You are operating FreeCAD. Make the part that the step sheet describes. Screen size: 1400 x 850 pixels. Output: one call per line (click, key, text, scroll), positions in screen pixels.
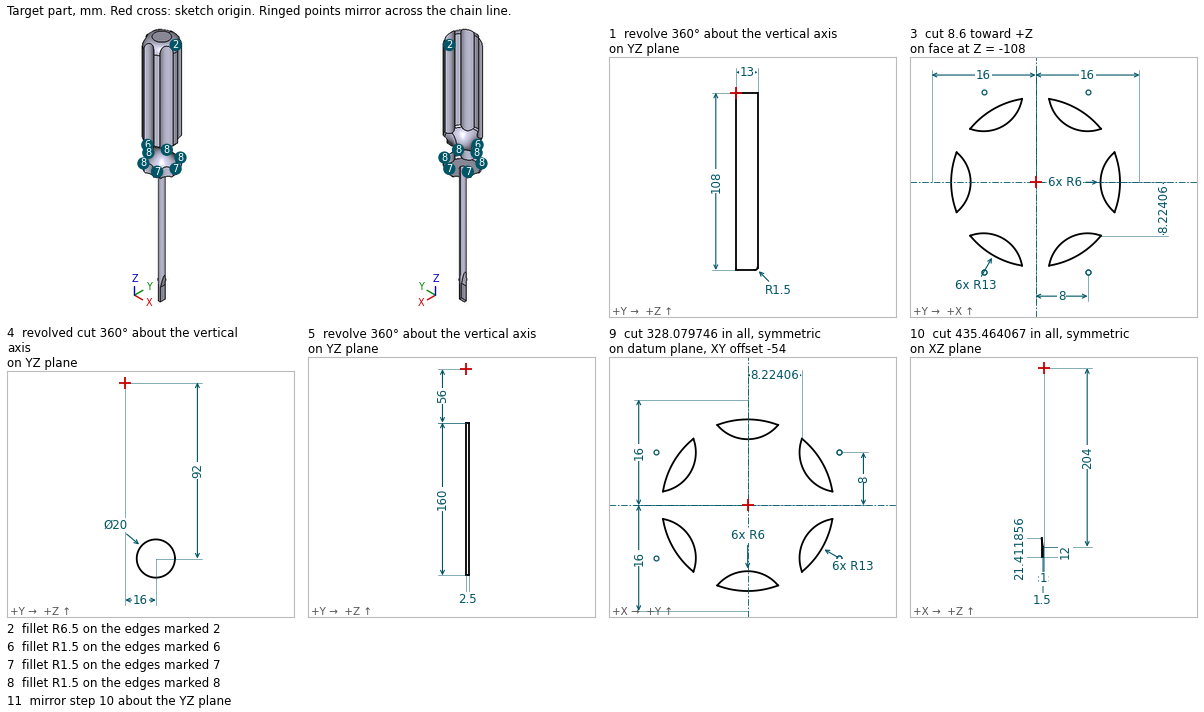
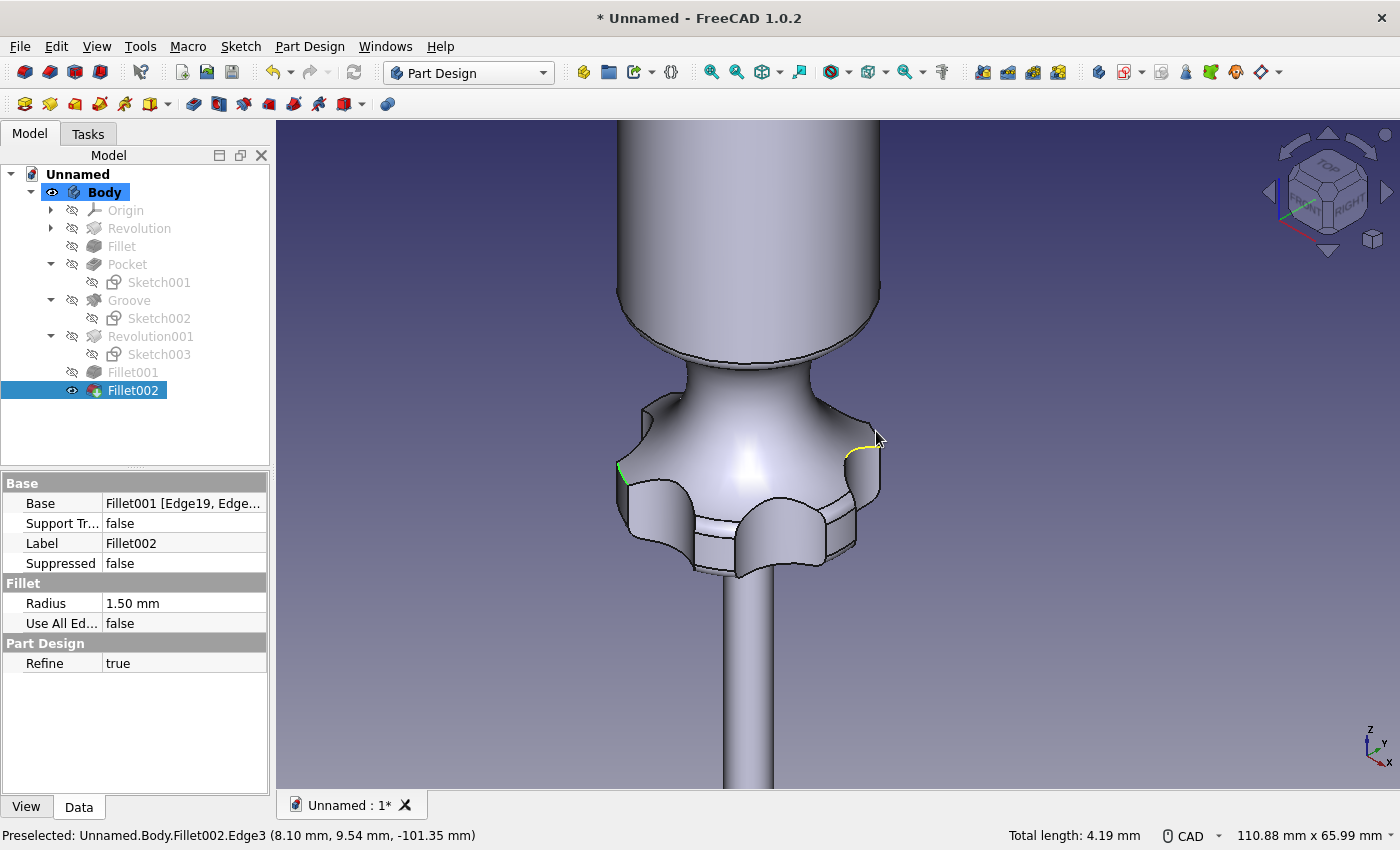
click(712, 72)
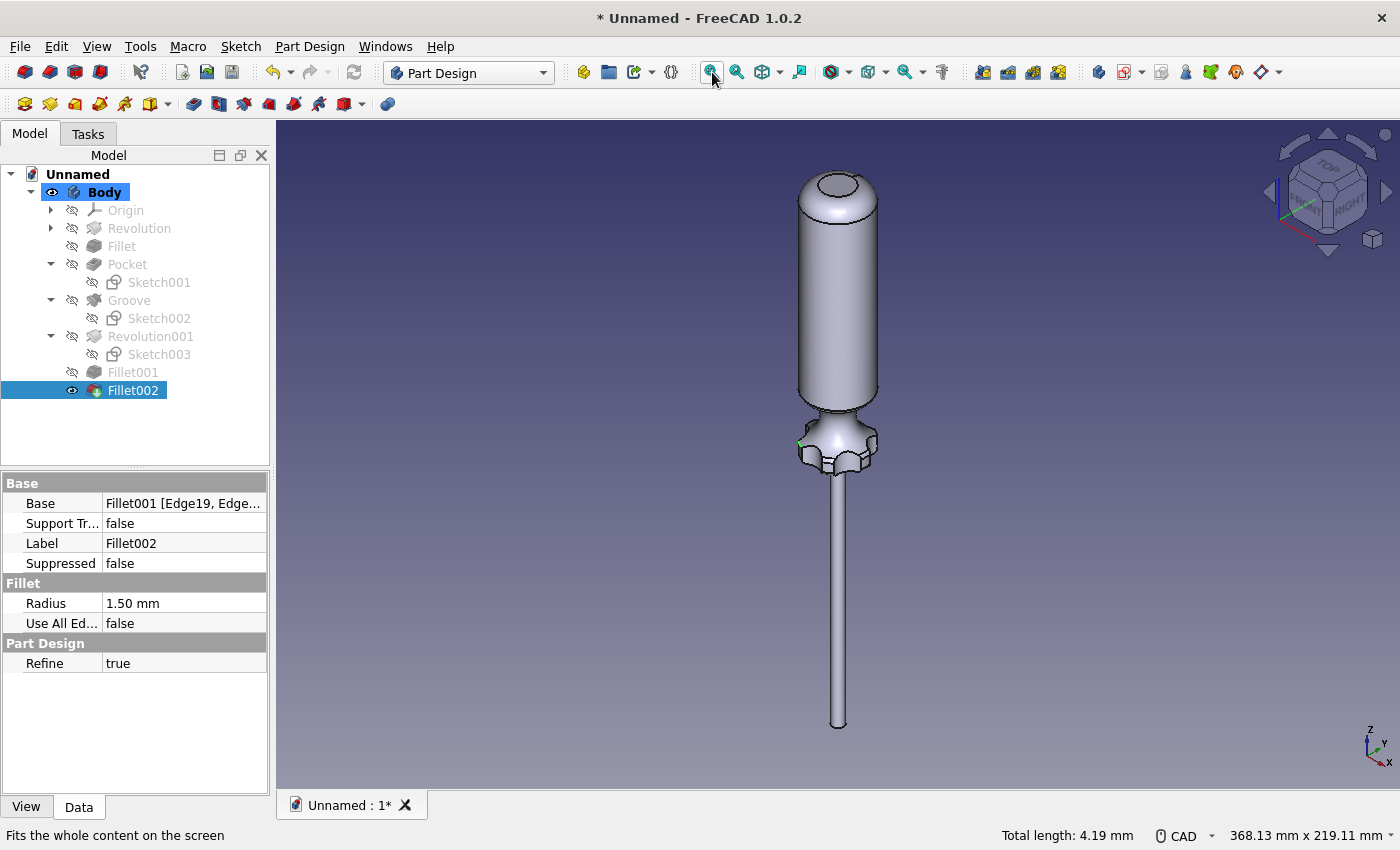
key(1)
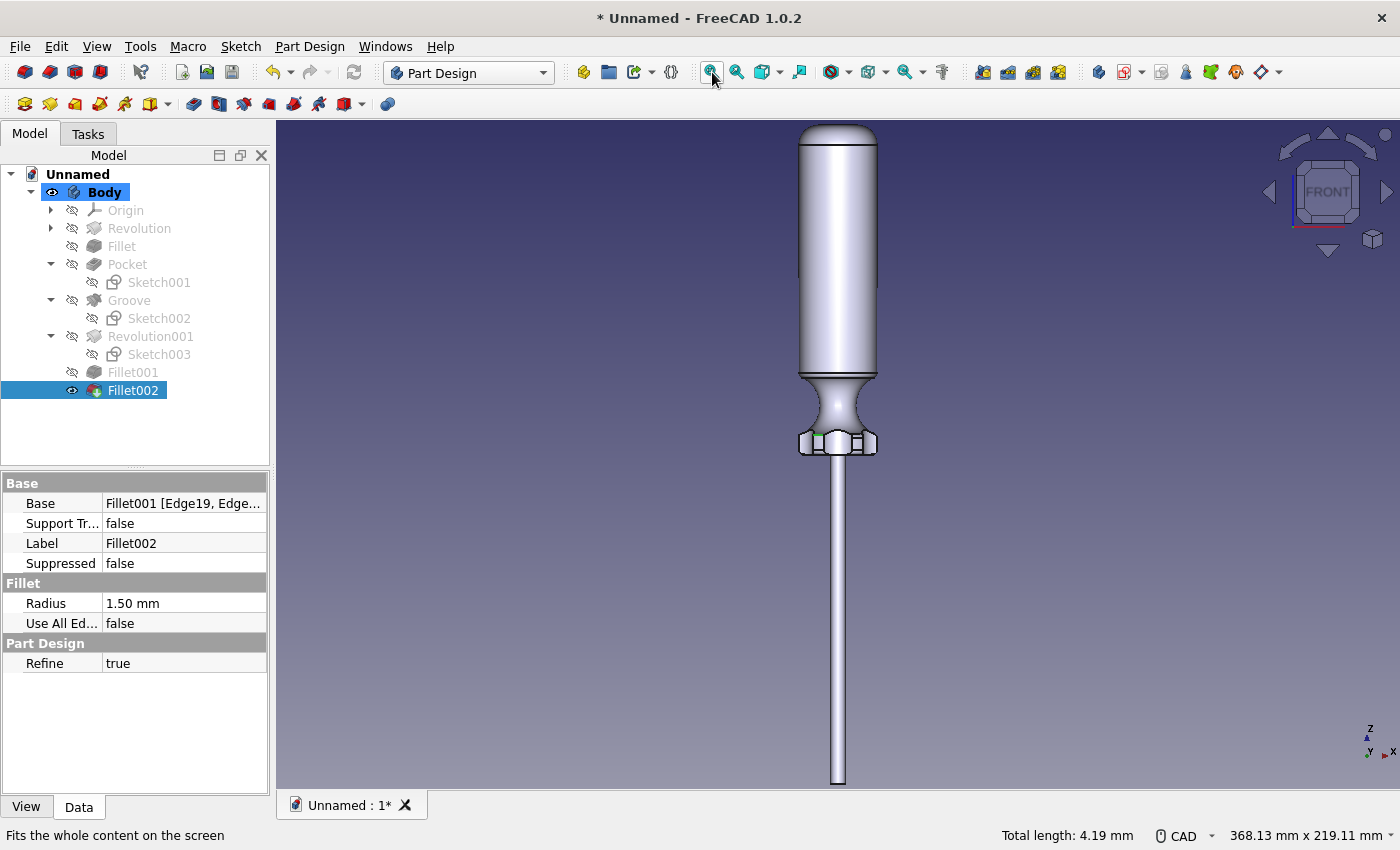
scroll(858, 434, up, 6)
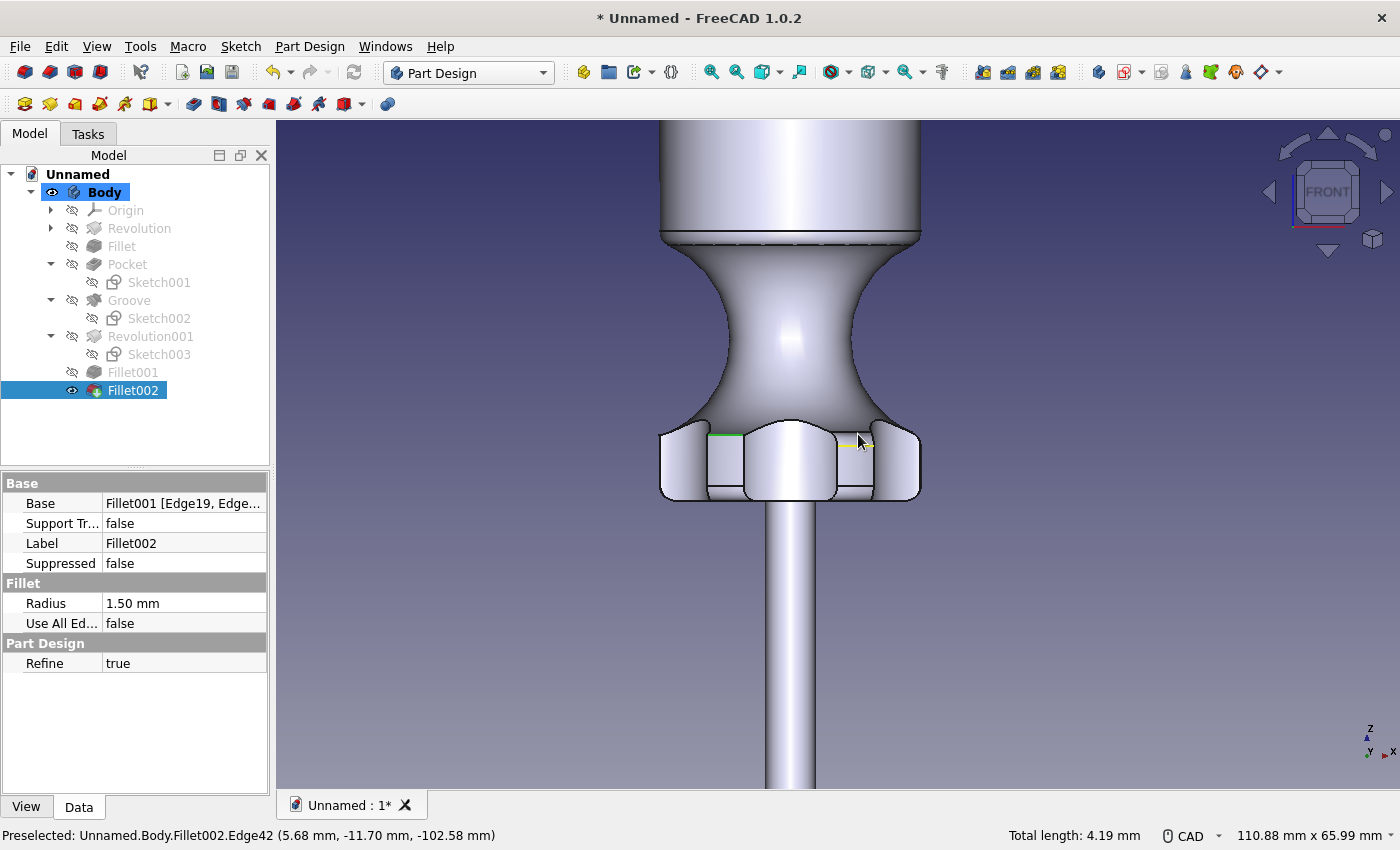
key(v)
key(f)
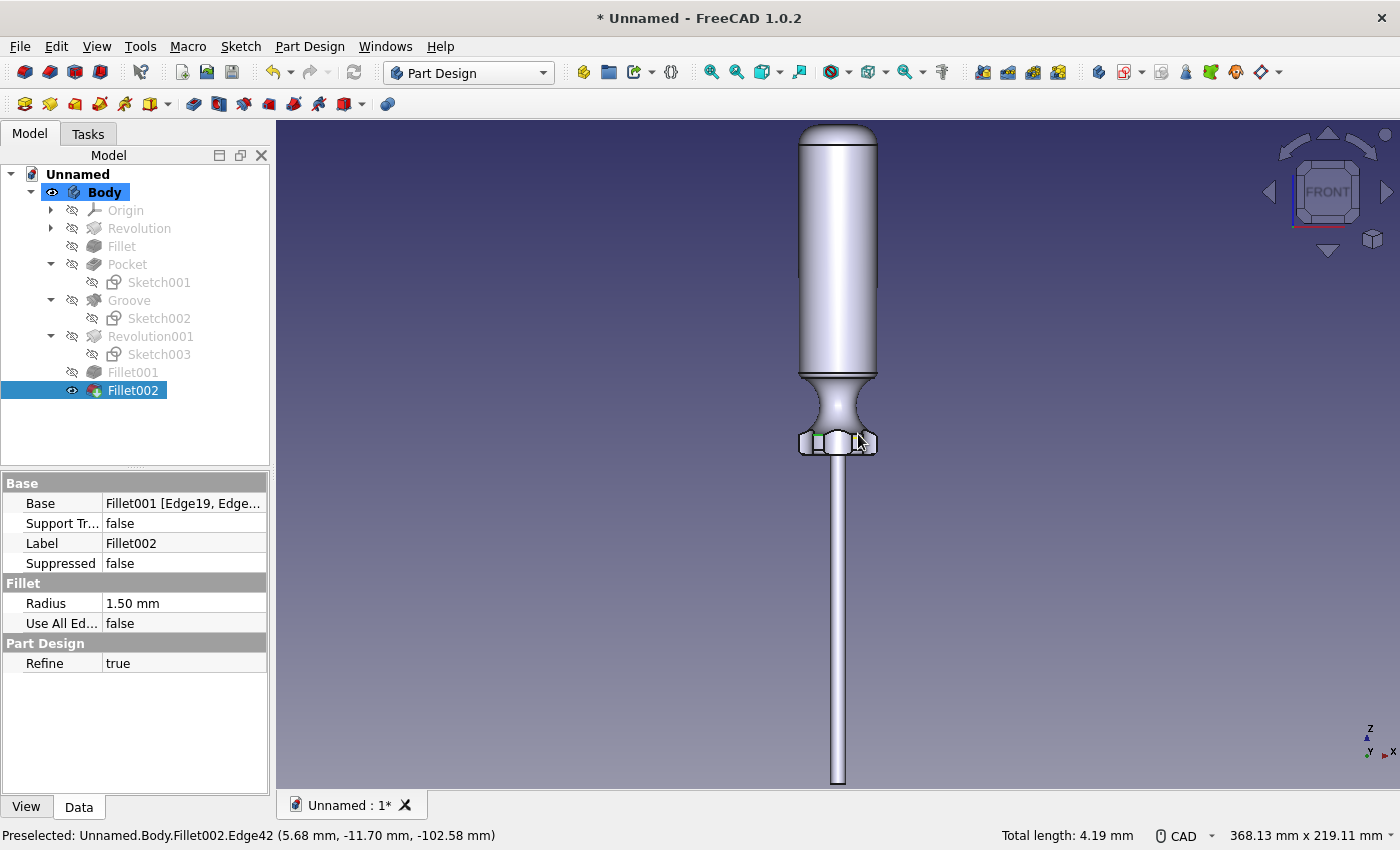
key(3)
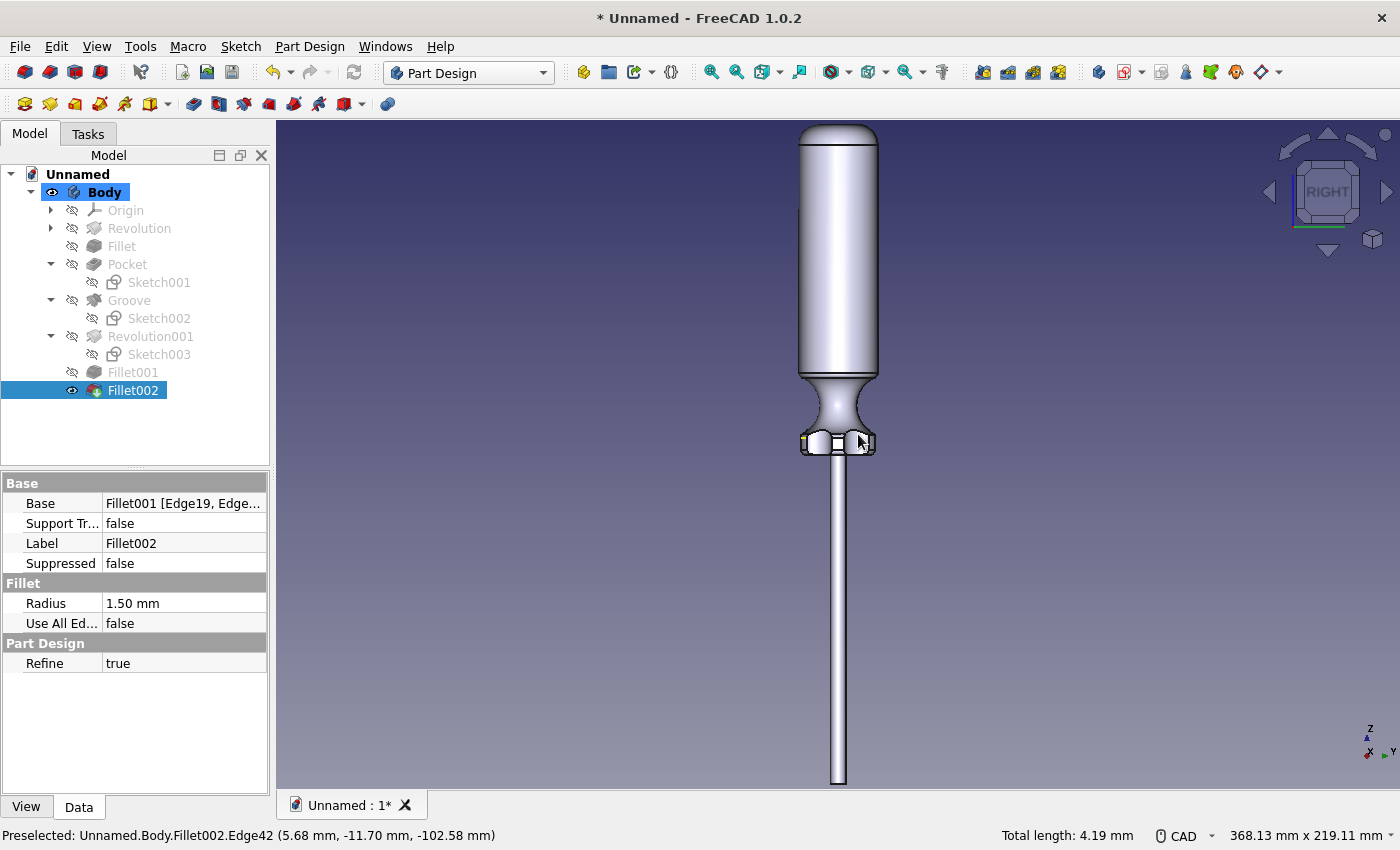
scroll(872, 434, up, 6)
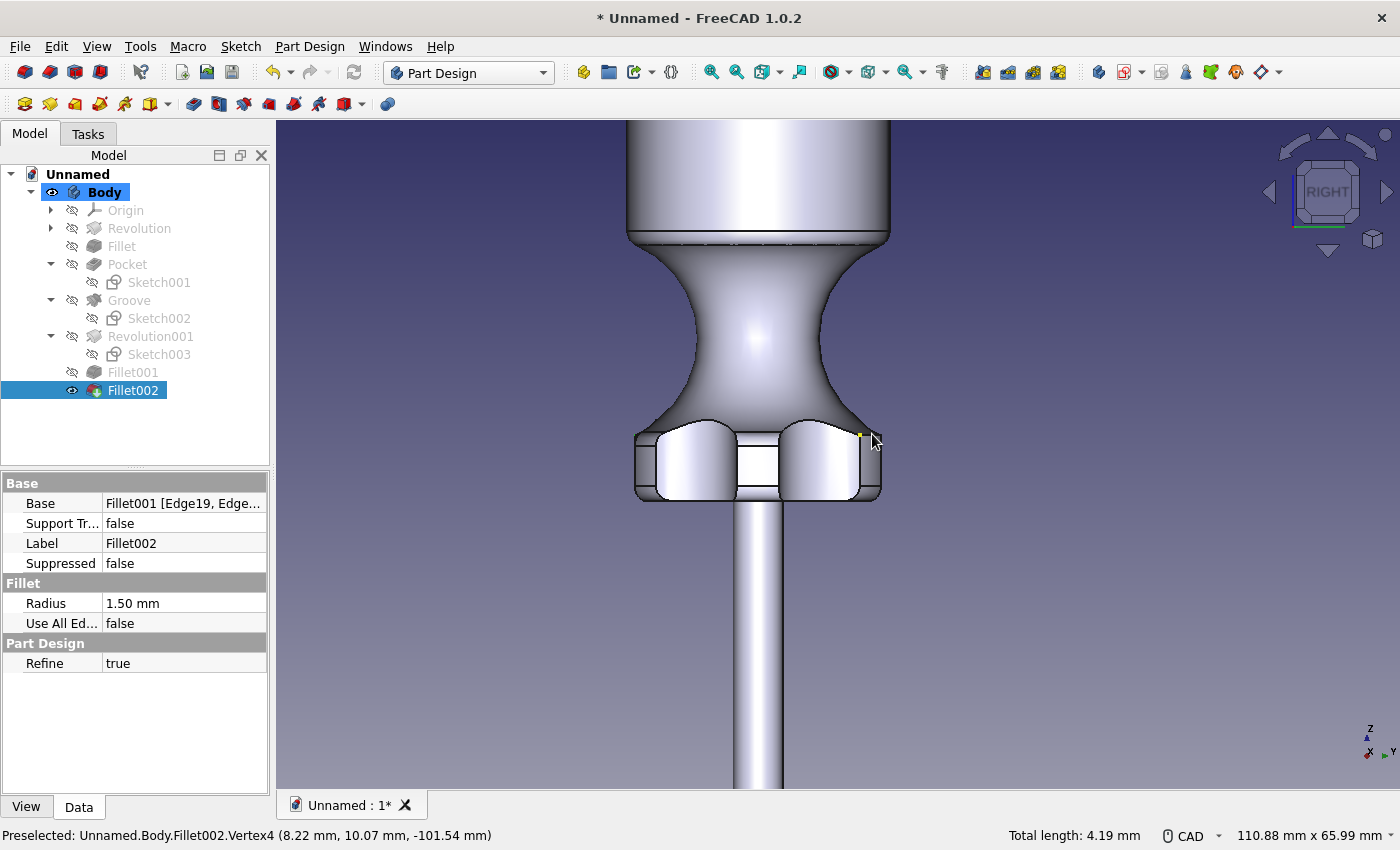
click(868, 434, ctrl)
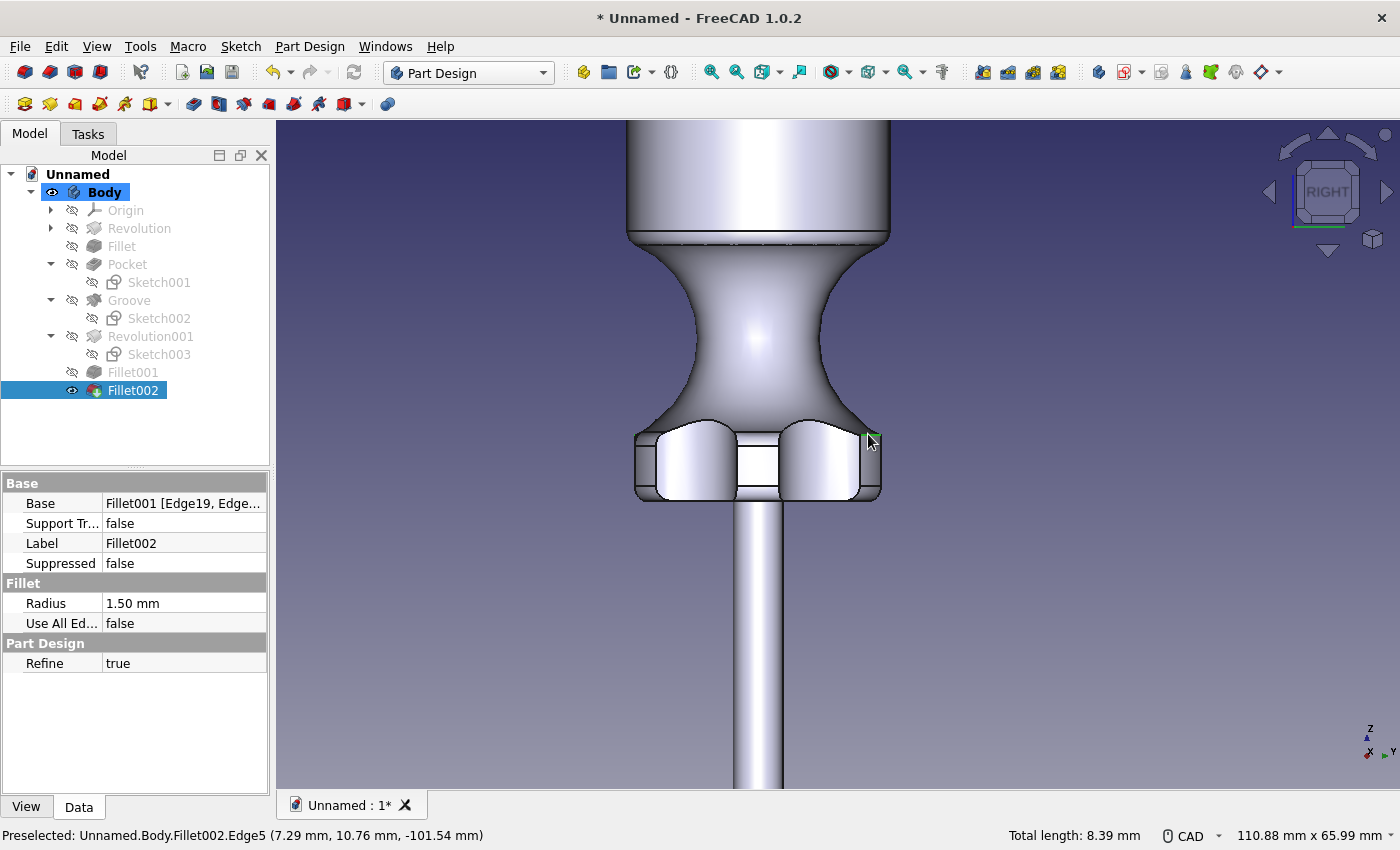
key(v)
key(f)